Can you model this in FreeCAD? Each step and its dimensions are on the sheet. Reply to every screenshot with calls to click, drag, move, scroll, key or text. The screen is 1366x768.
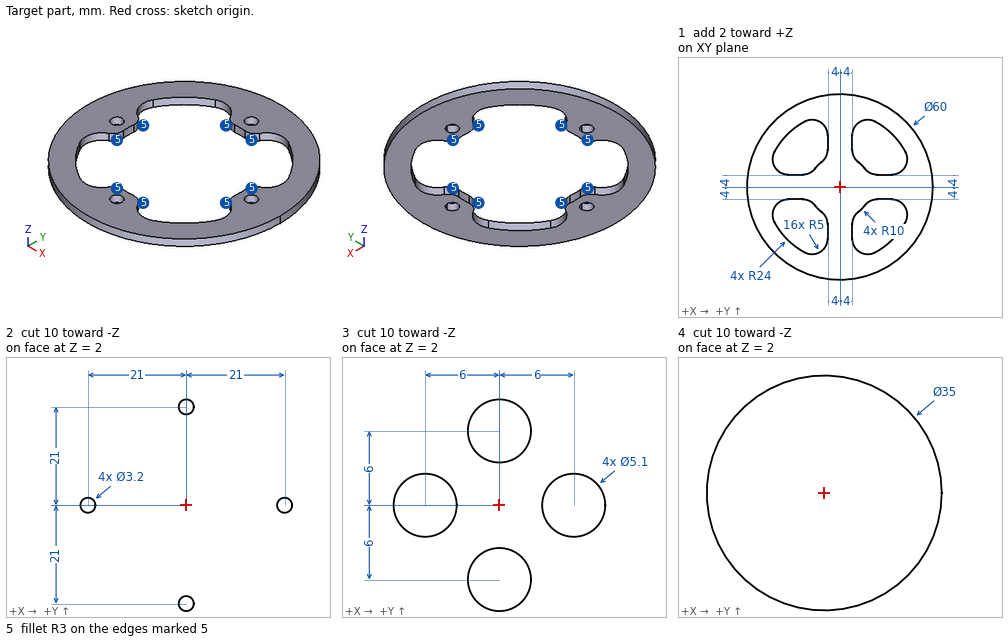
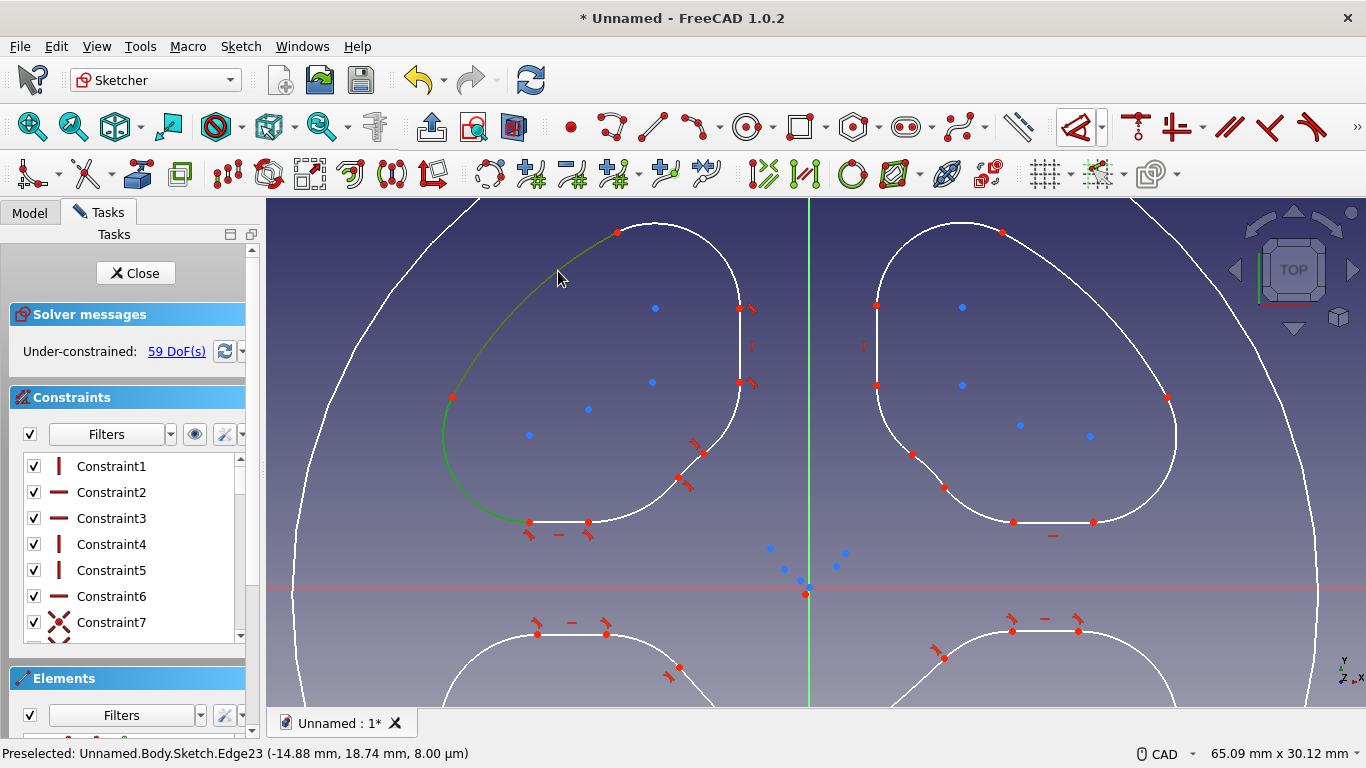
click(1312, 128)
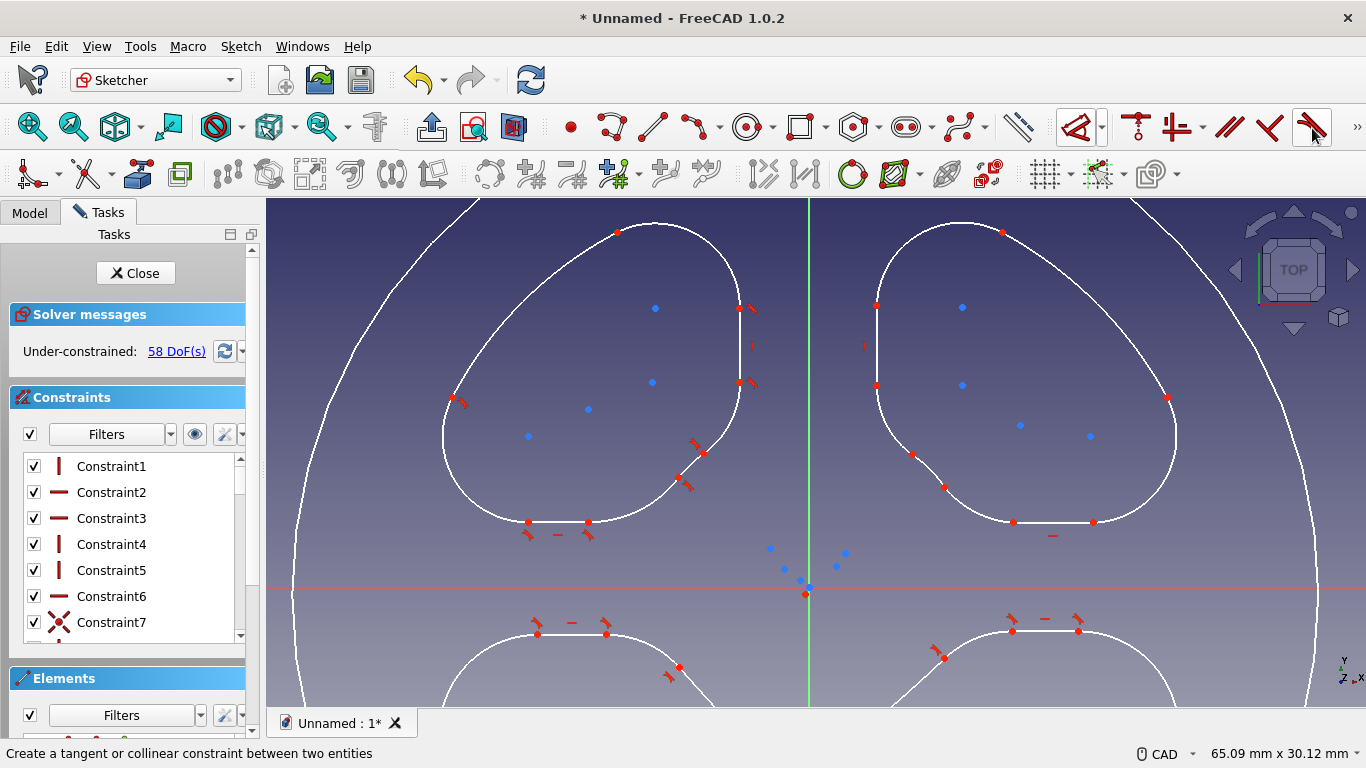
click(558, 271)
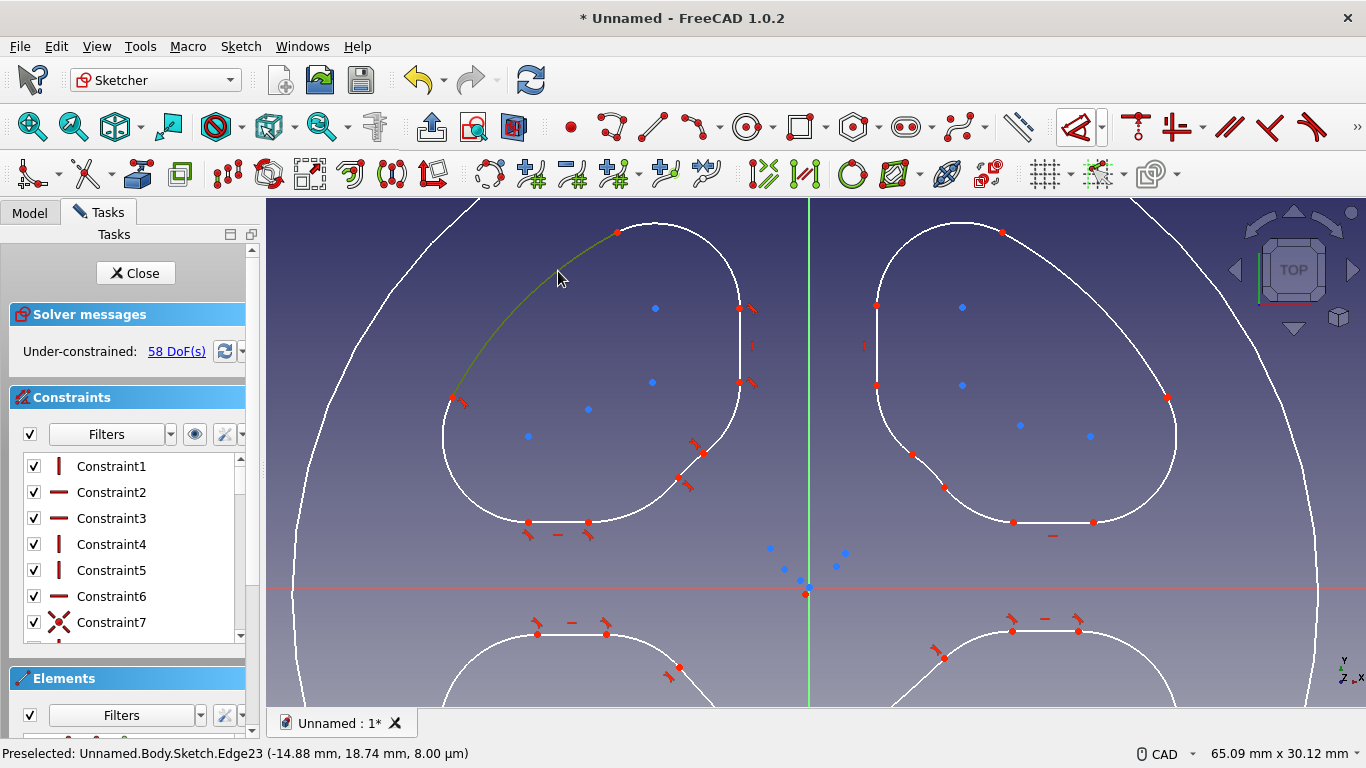
click(725, 260)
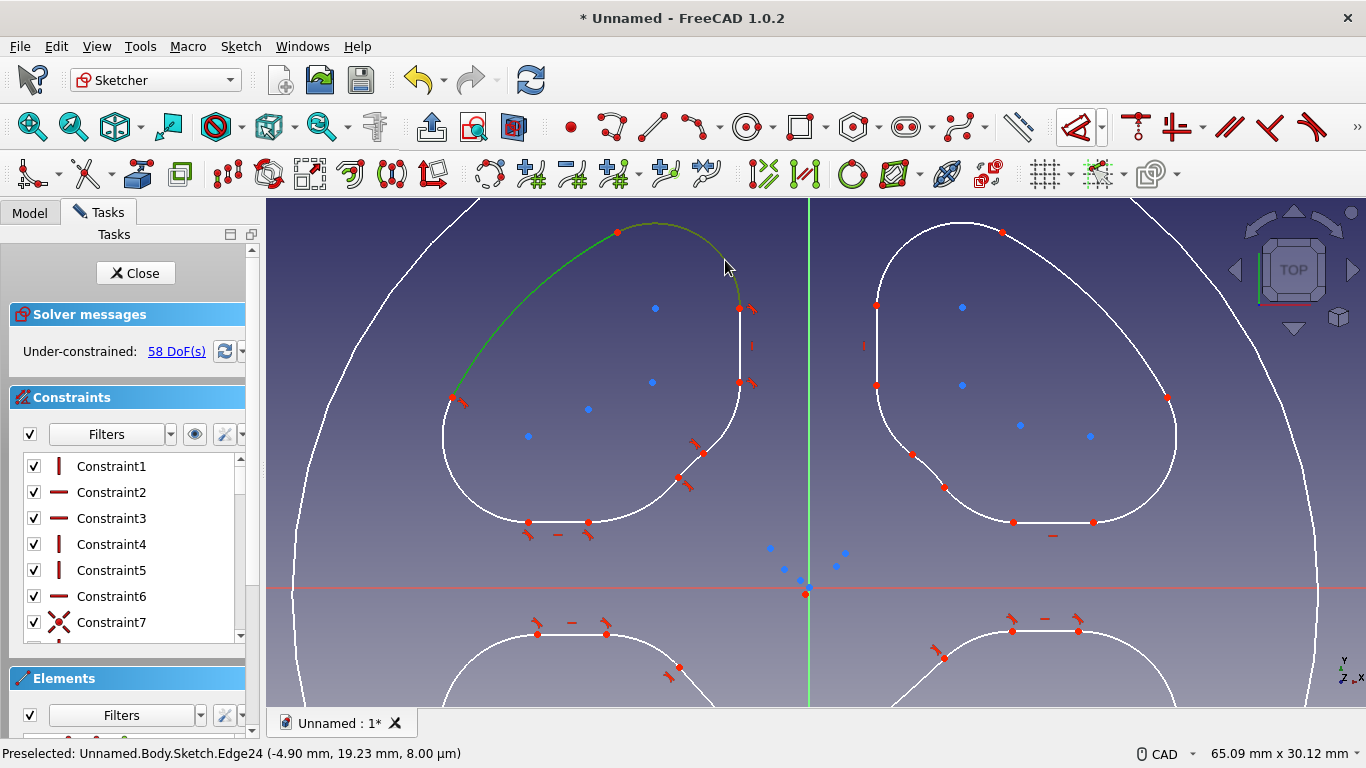
key(t)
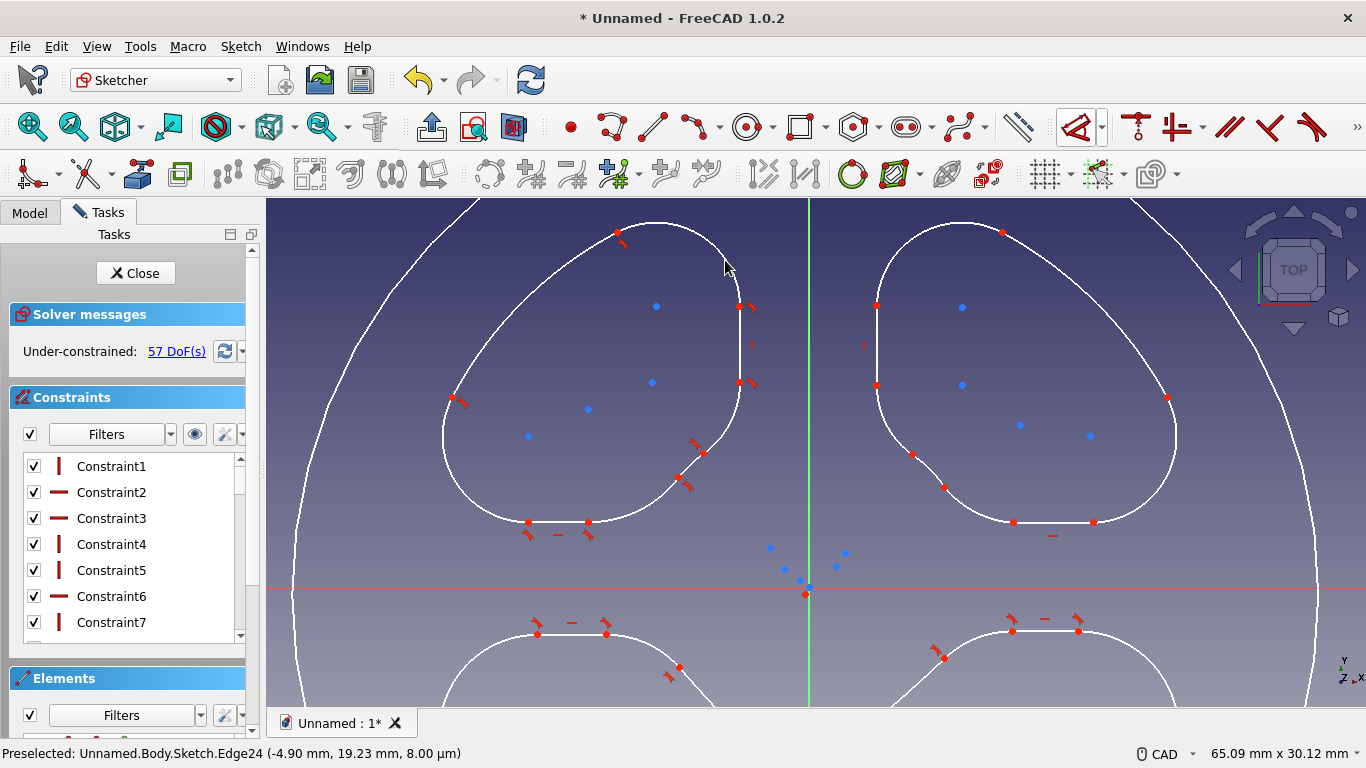
click(877, 362)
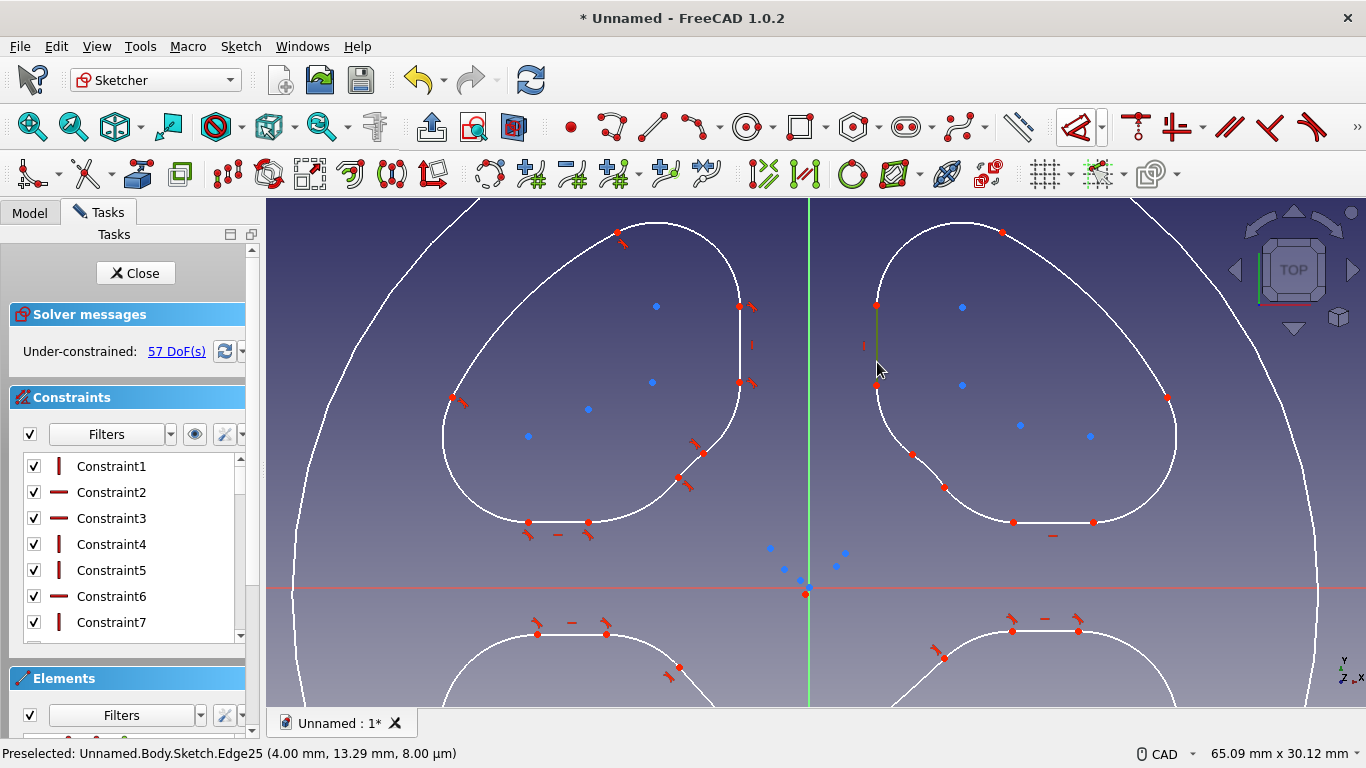
click(894, 257)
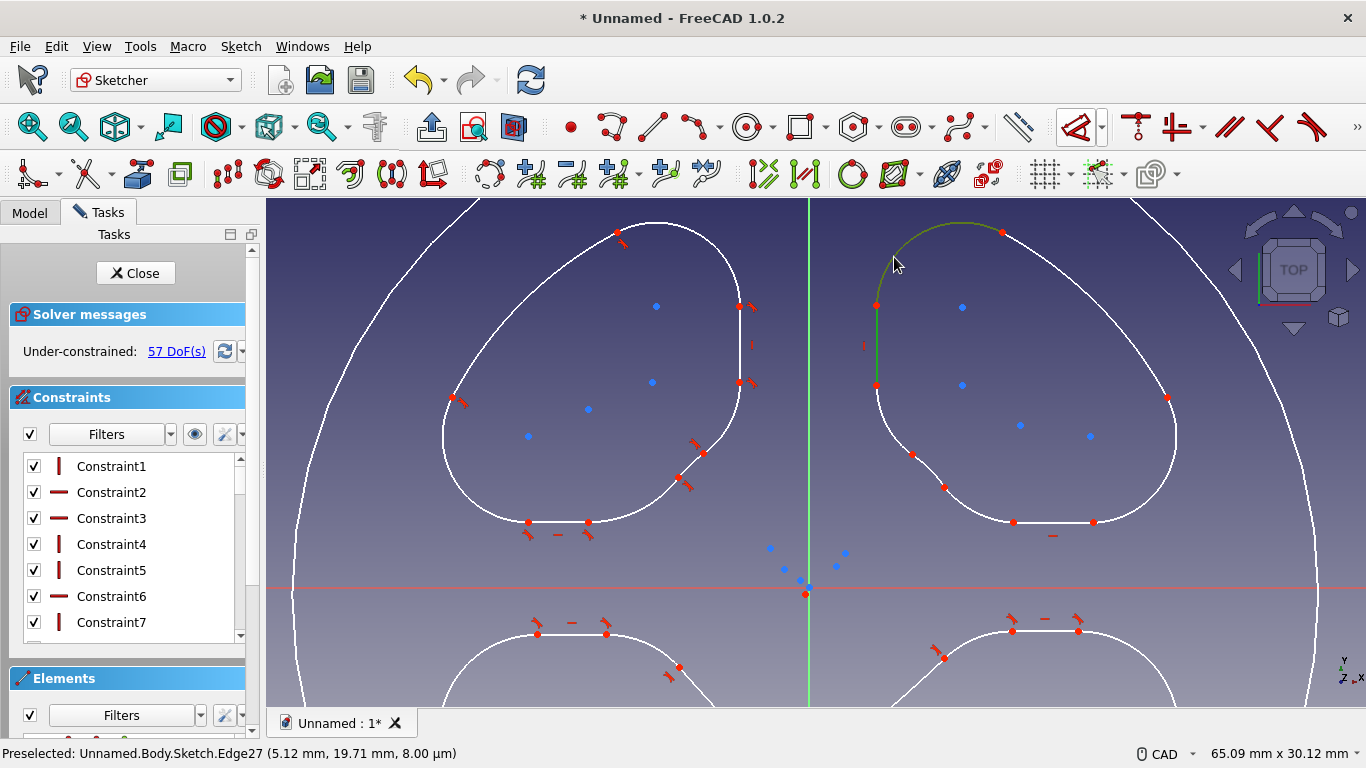
key(t)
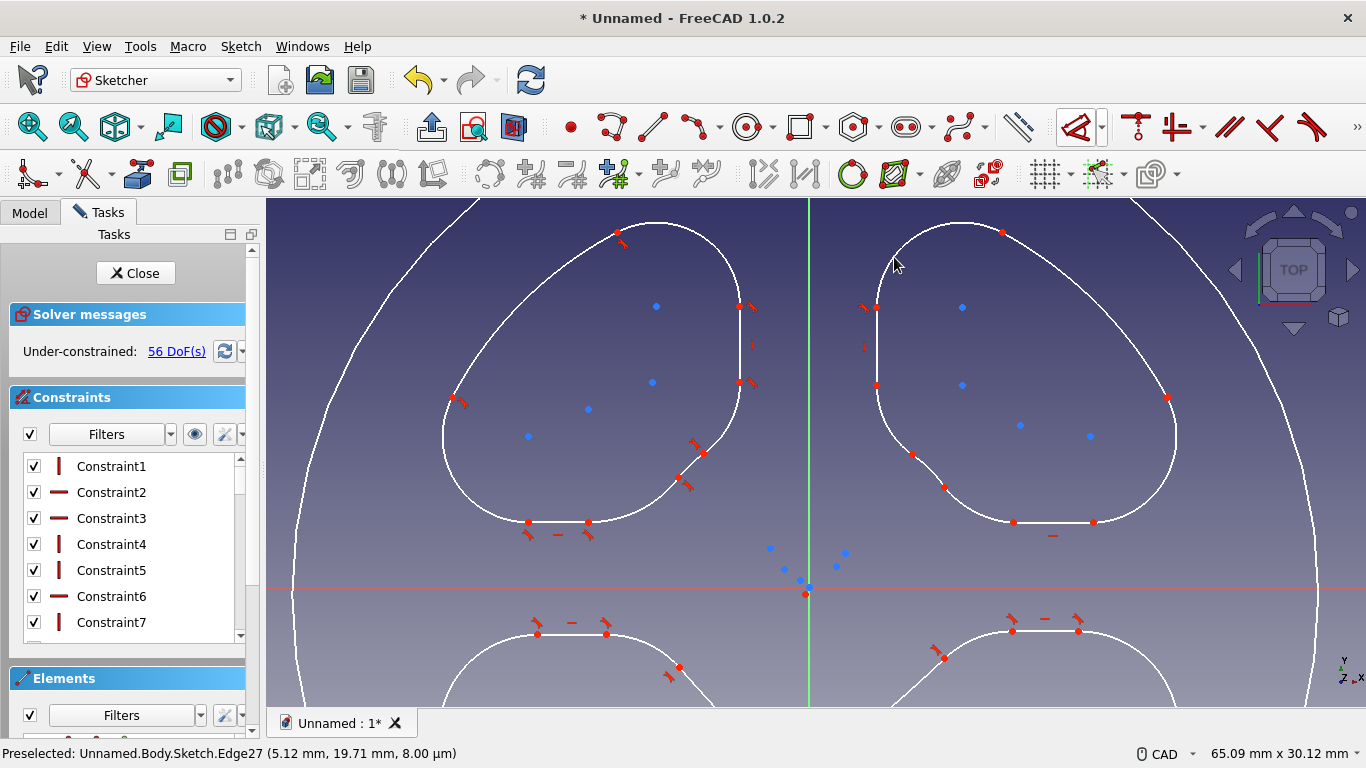
click(877, 362)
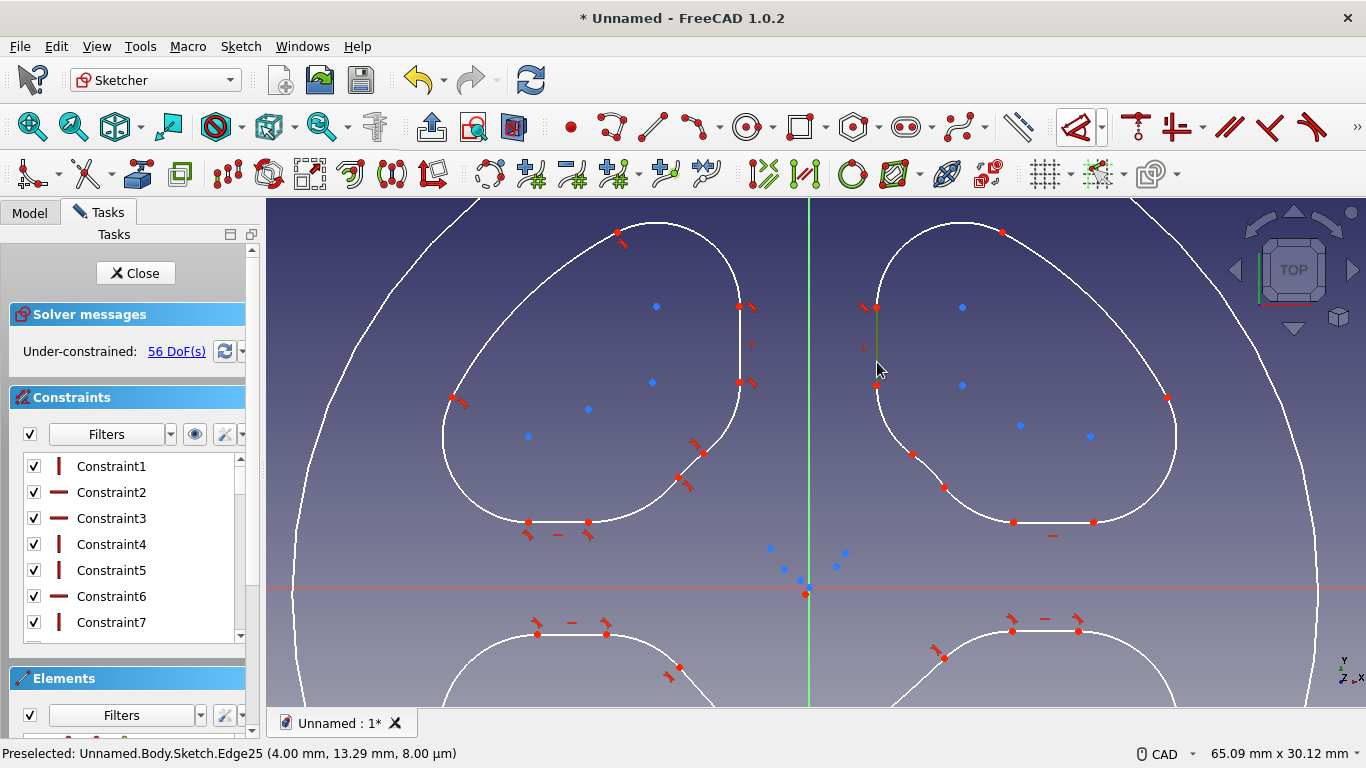
click(880, 410)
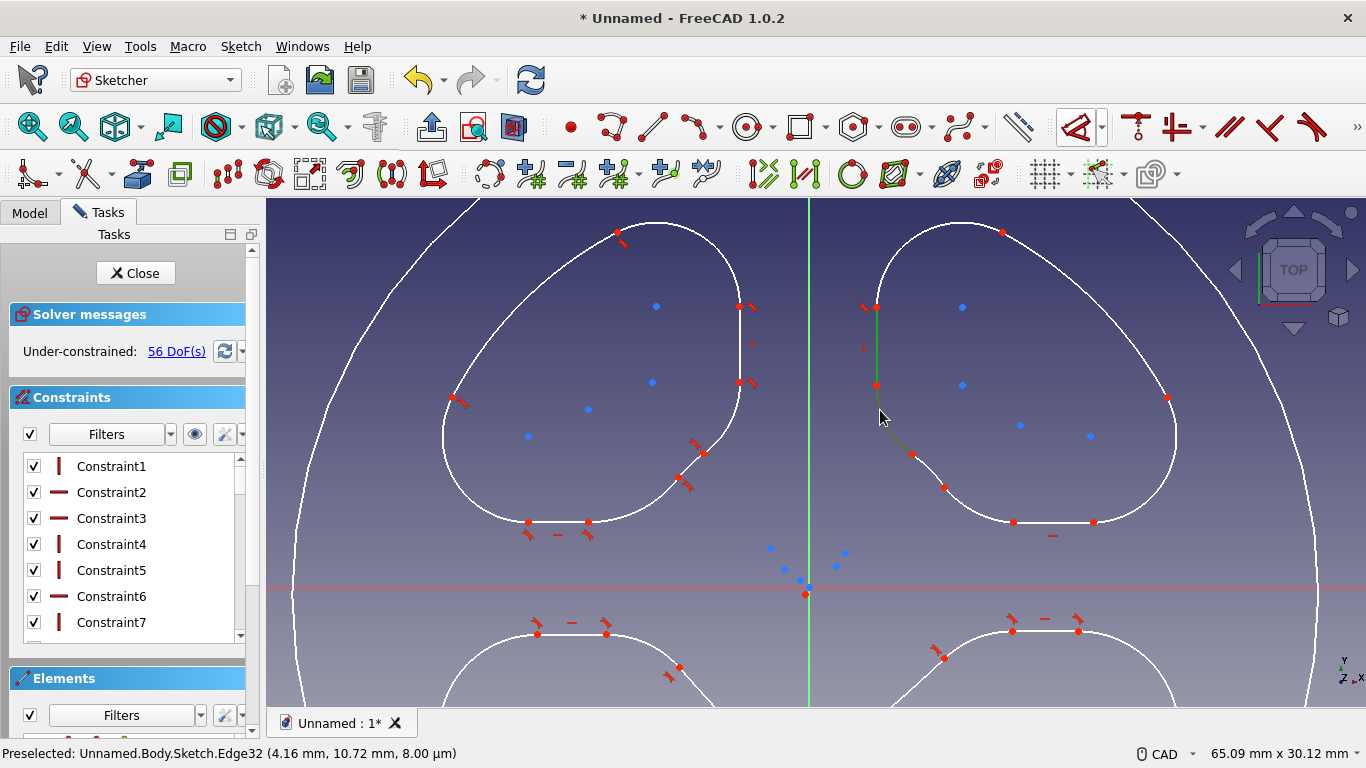
key(t)